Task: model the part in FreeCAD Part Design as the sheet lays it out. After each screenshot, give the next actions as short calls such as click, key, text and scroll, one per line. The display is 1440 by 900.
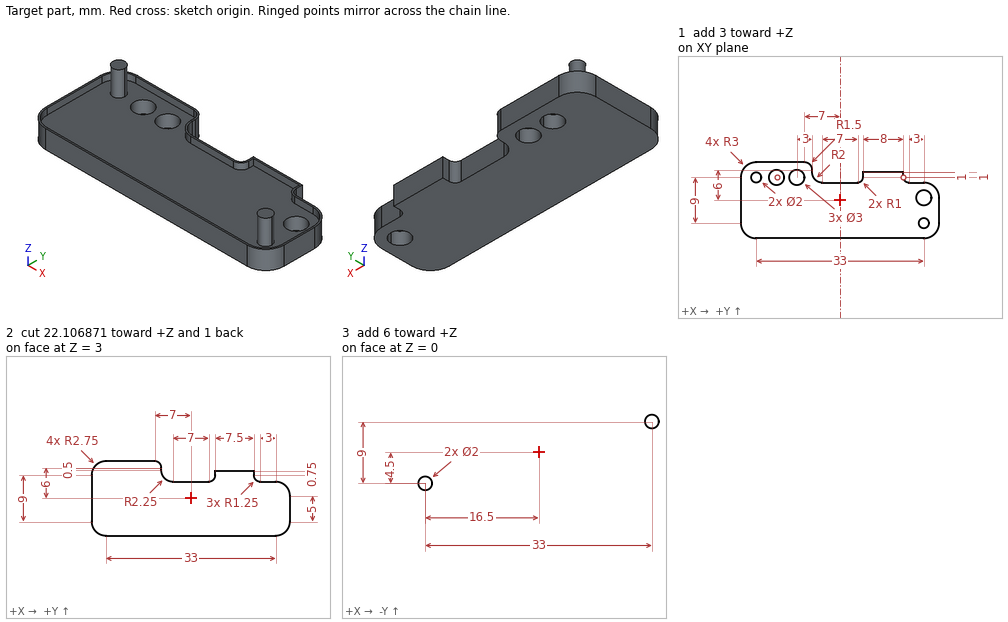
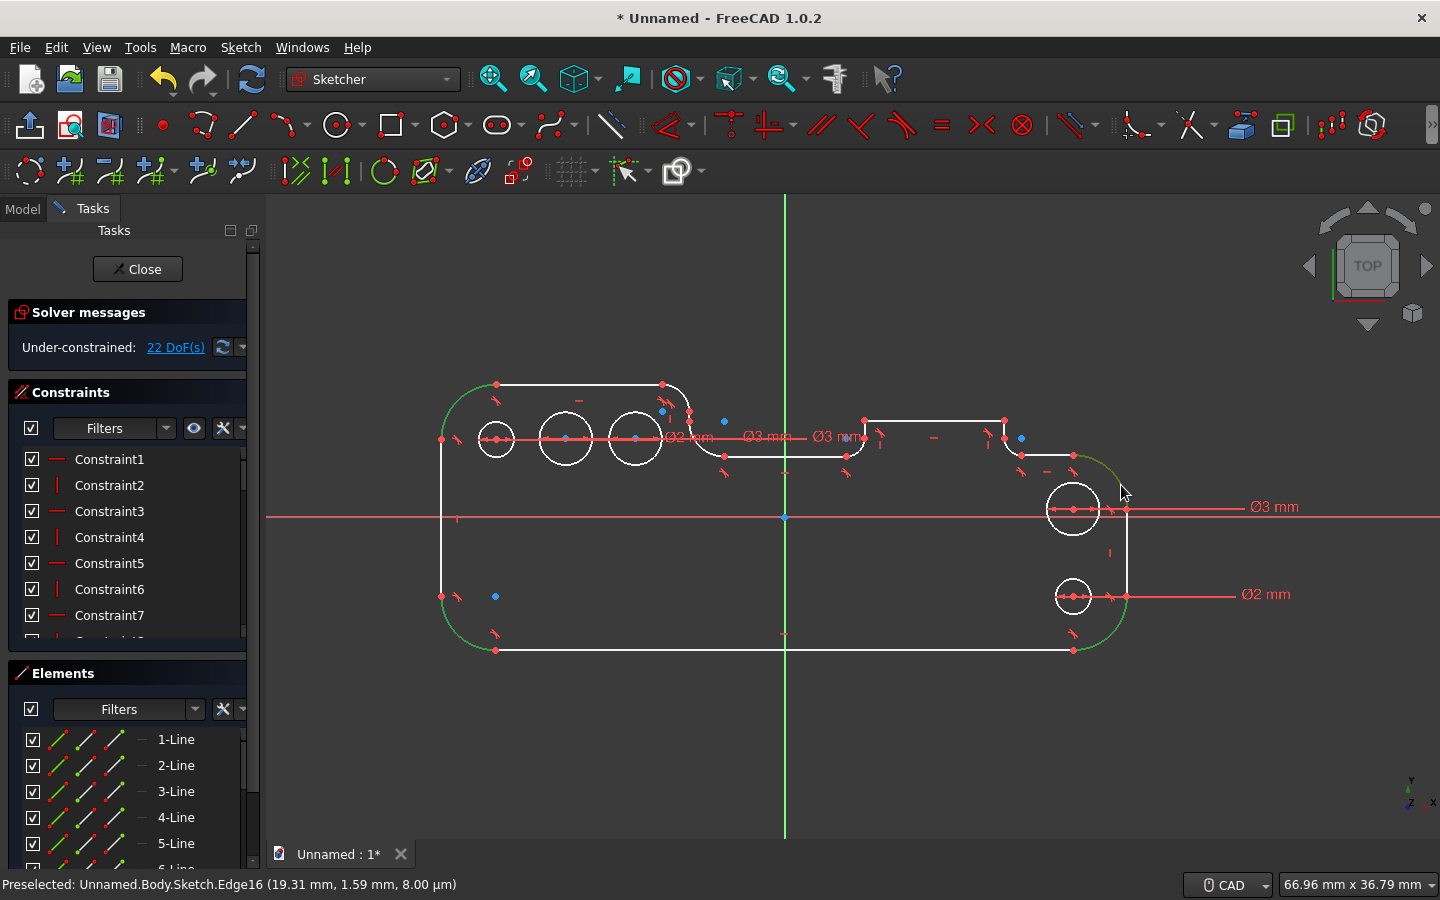
click(942, 126)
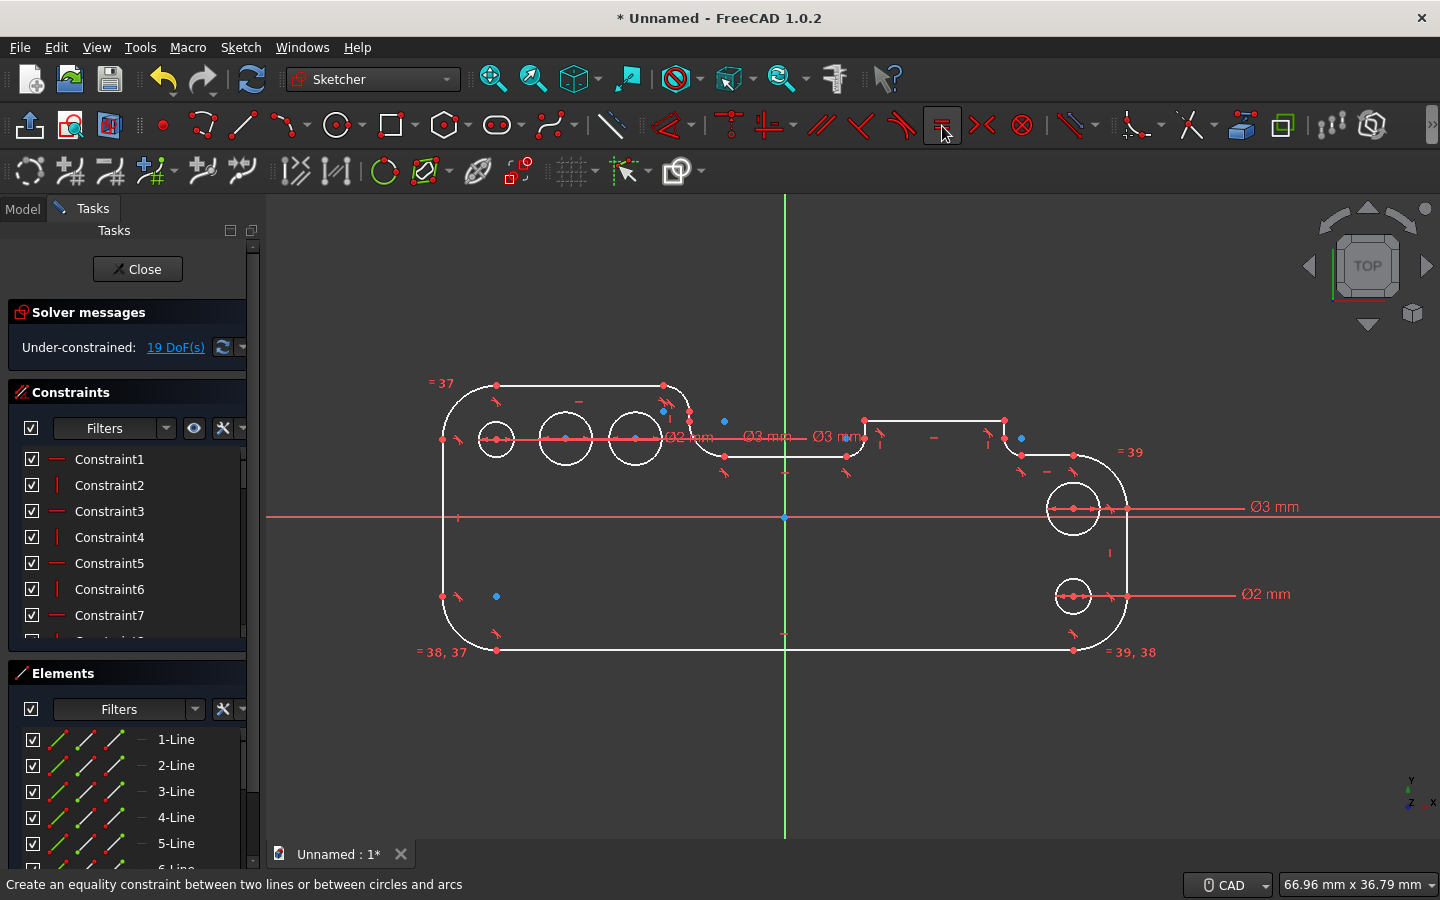
click(1009, 450)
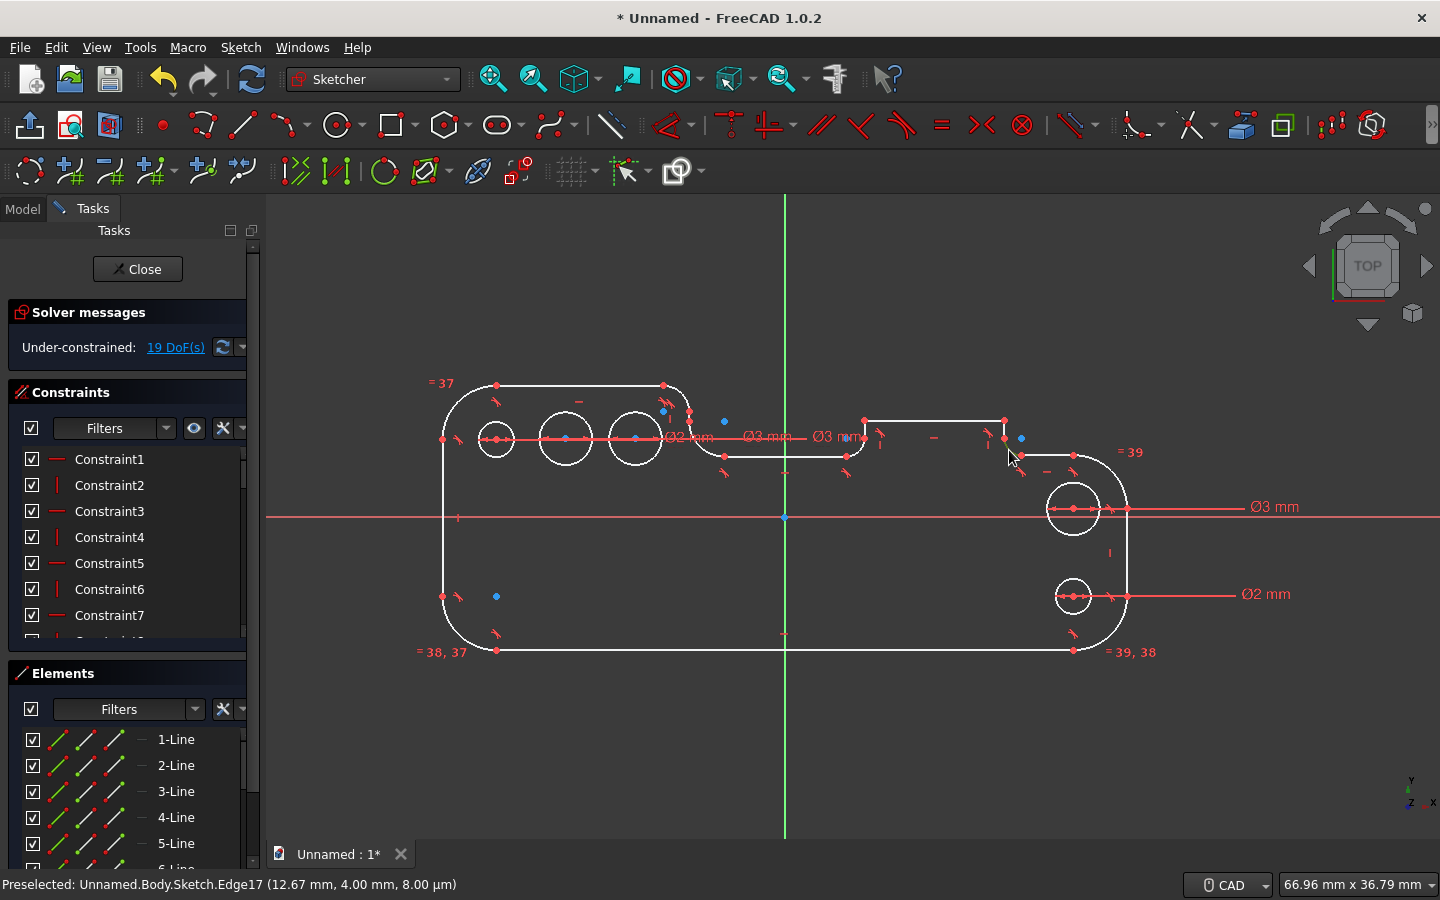
click(859, 451)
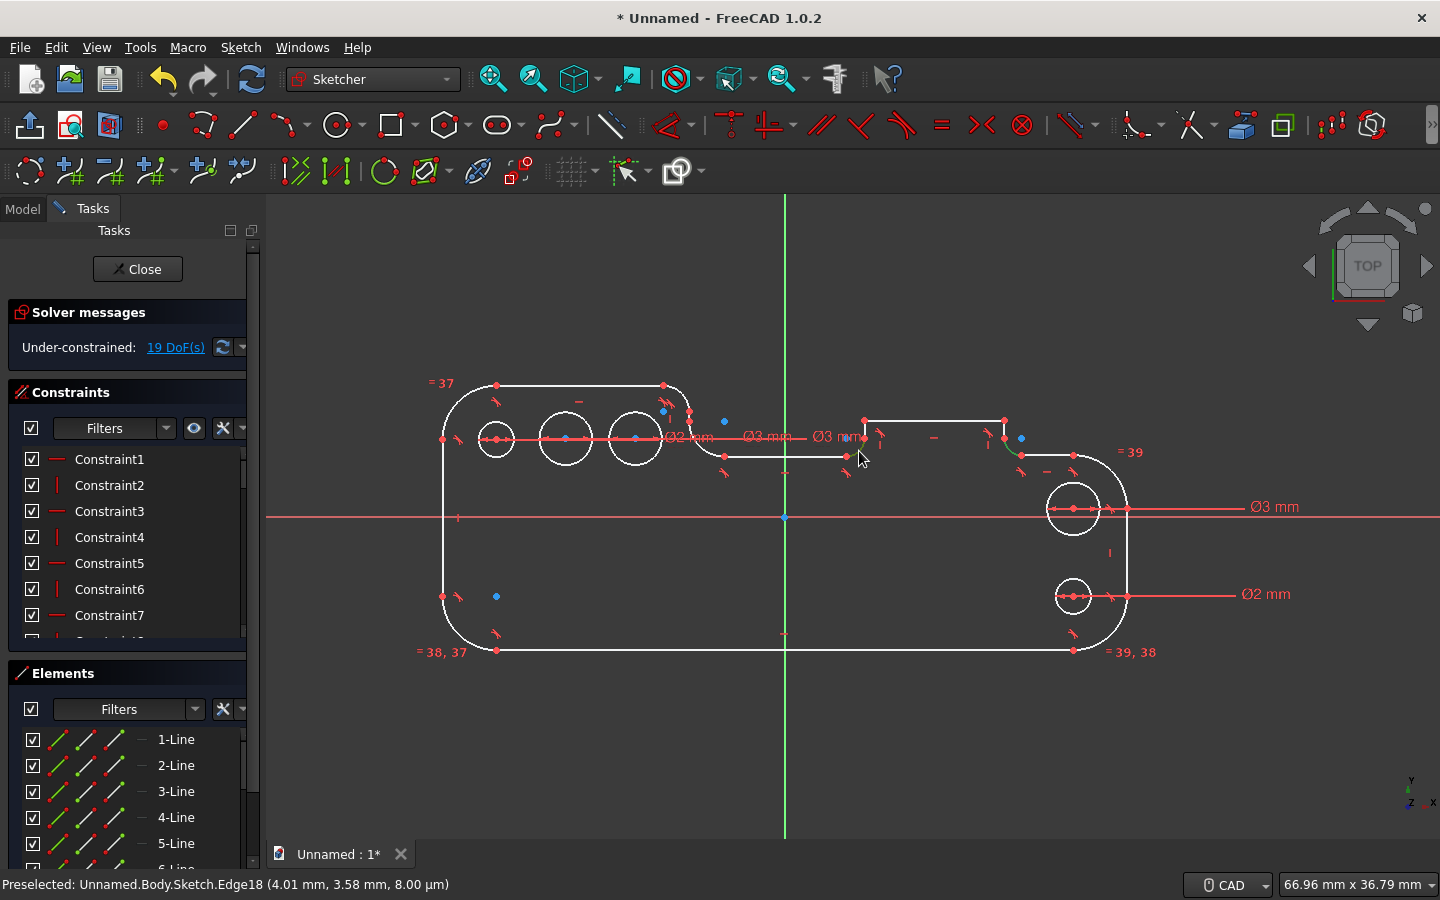
click(942, 126)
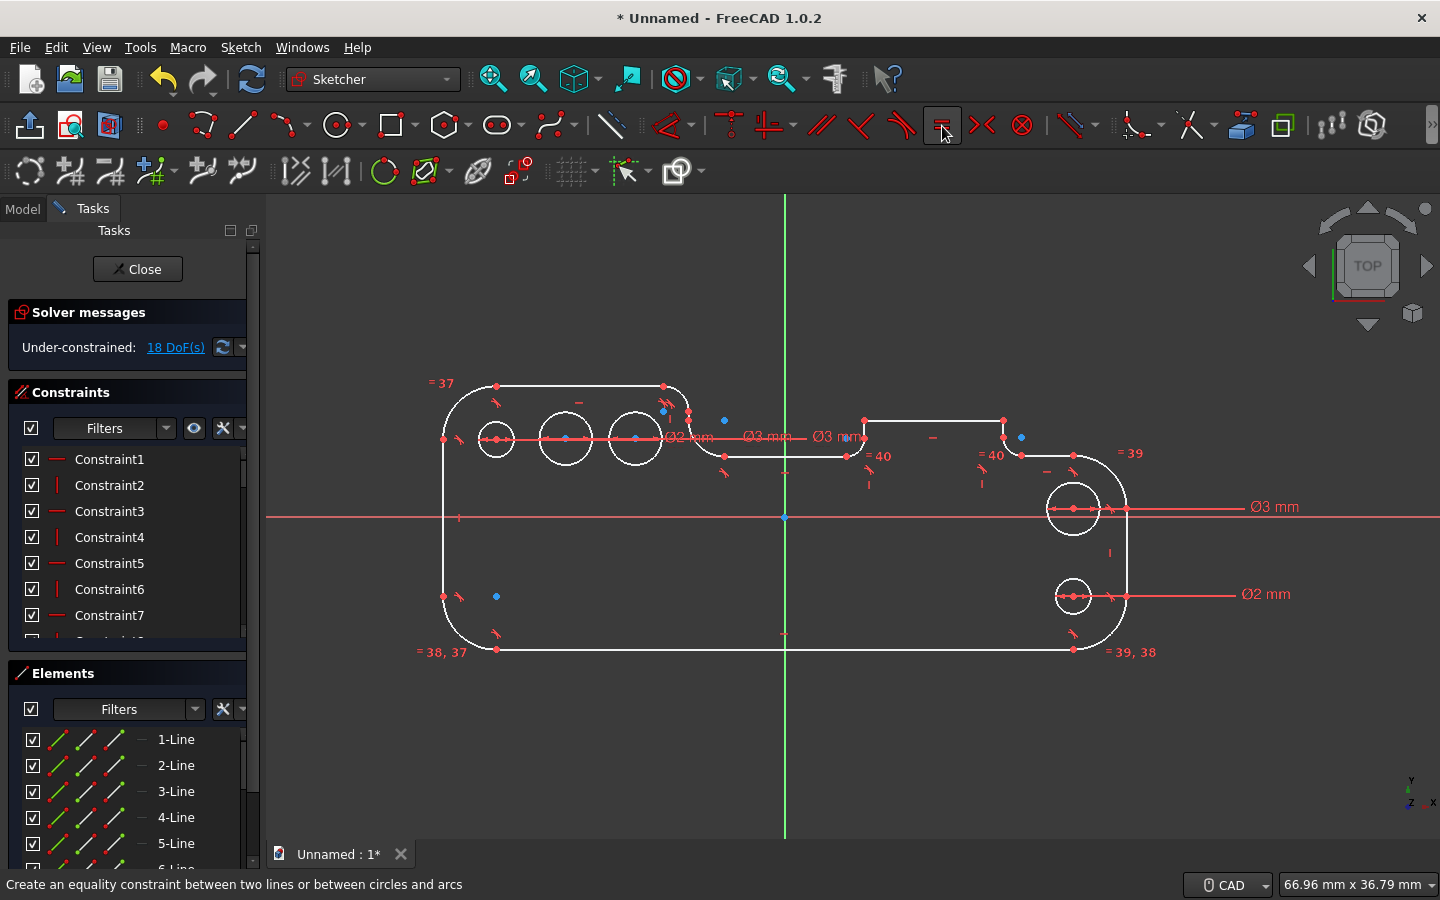
click(635, 439)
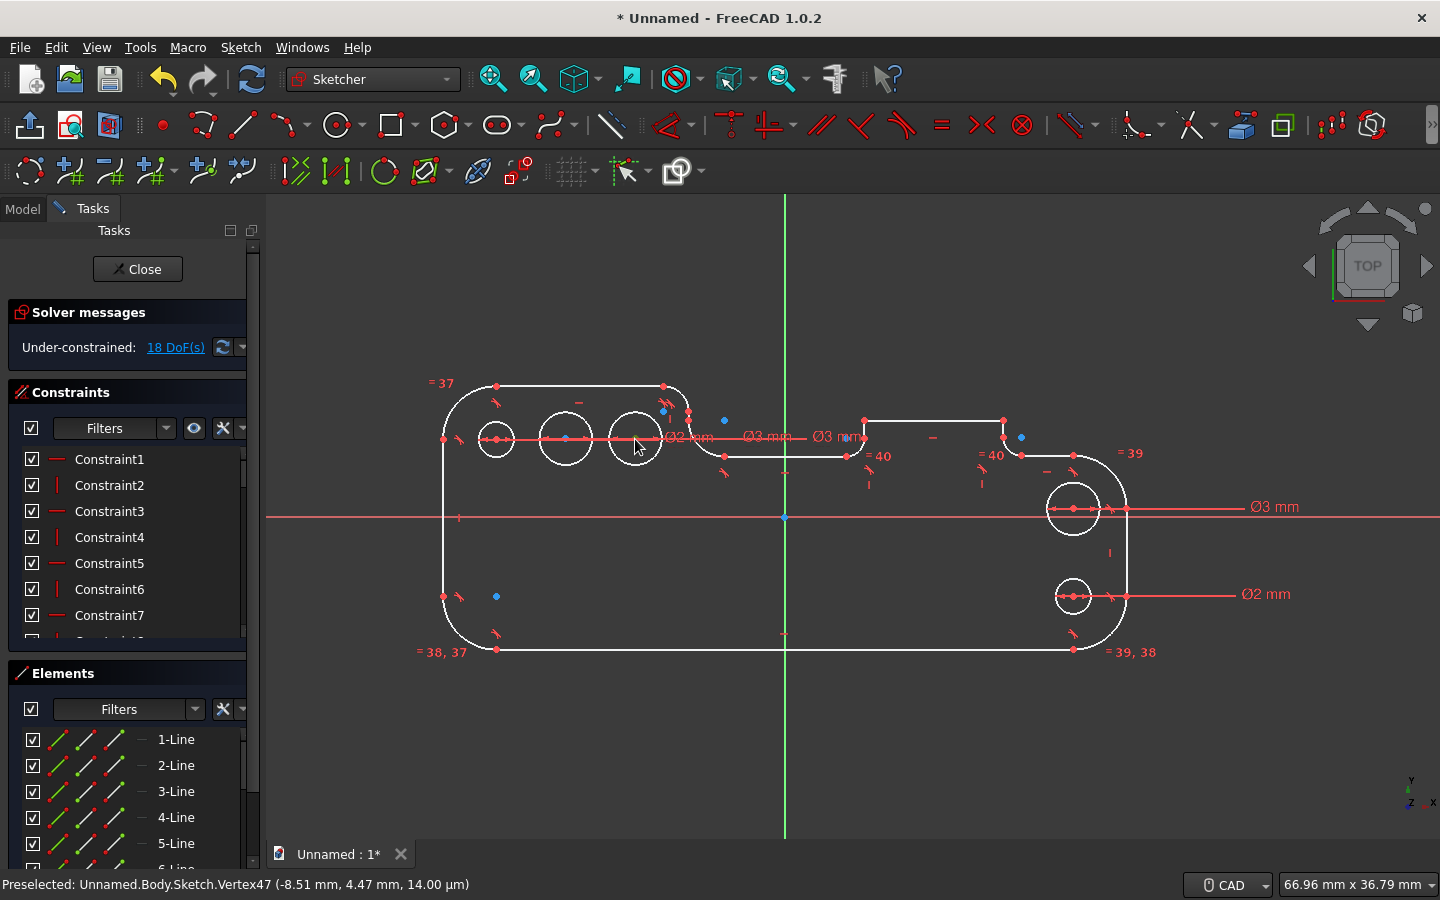
click(566, 439)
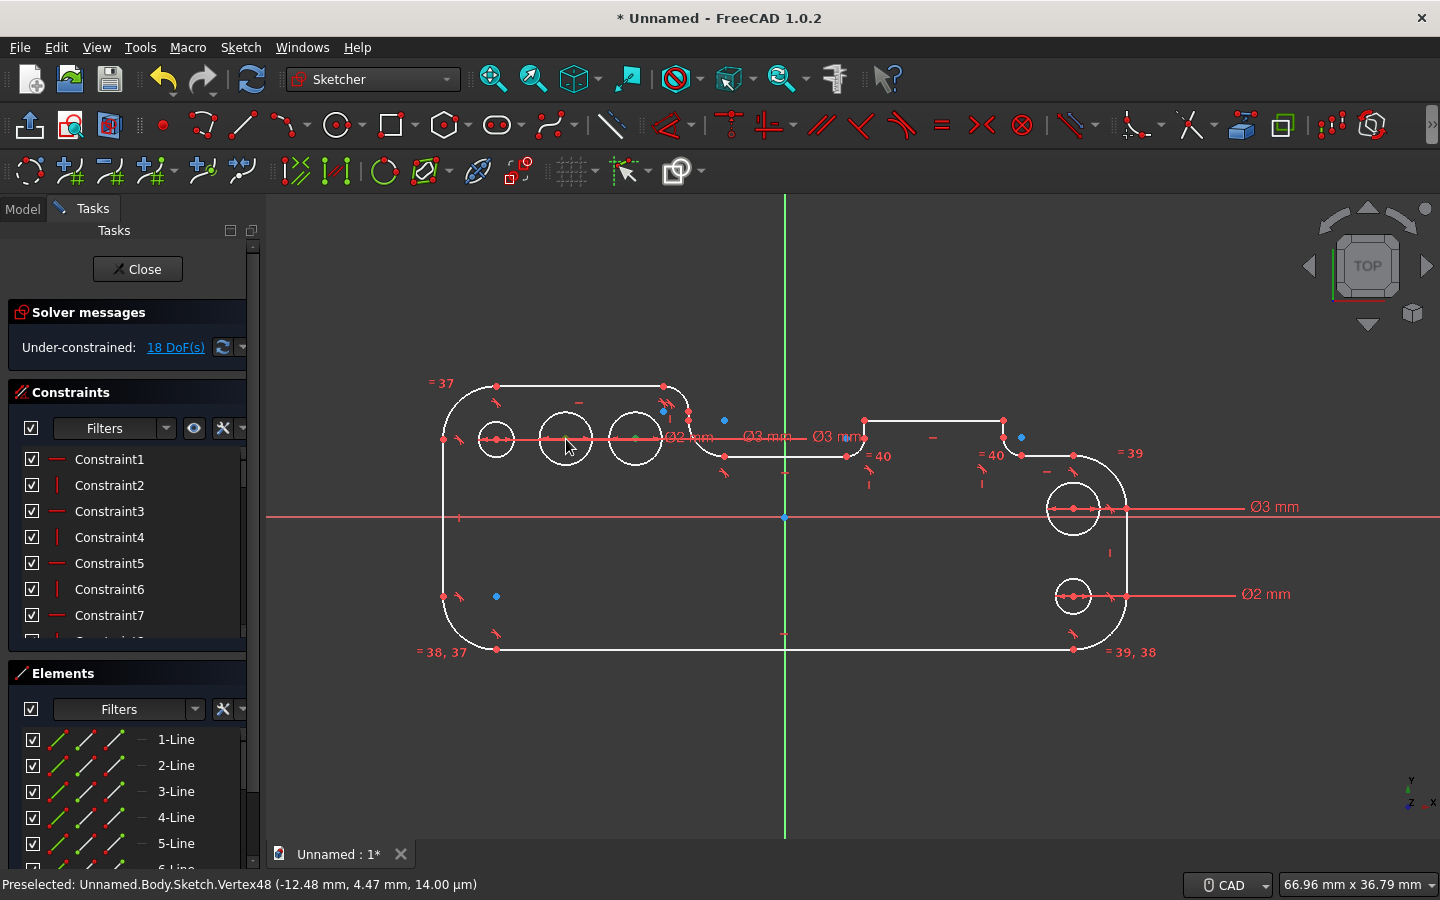
click(796, 126)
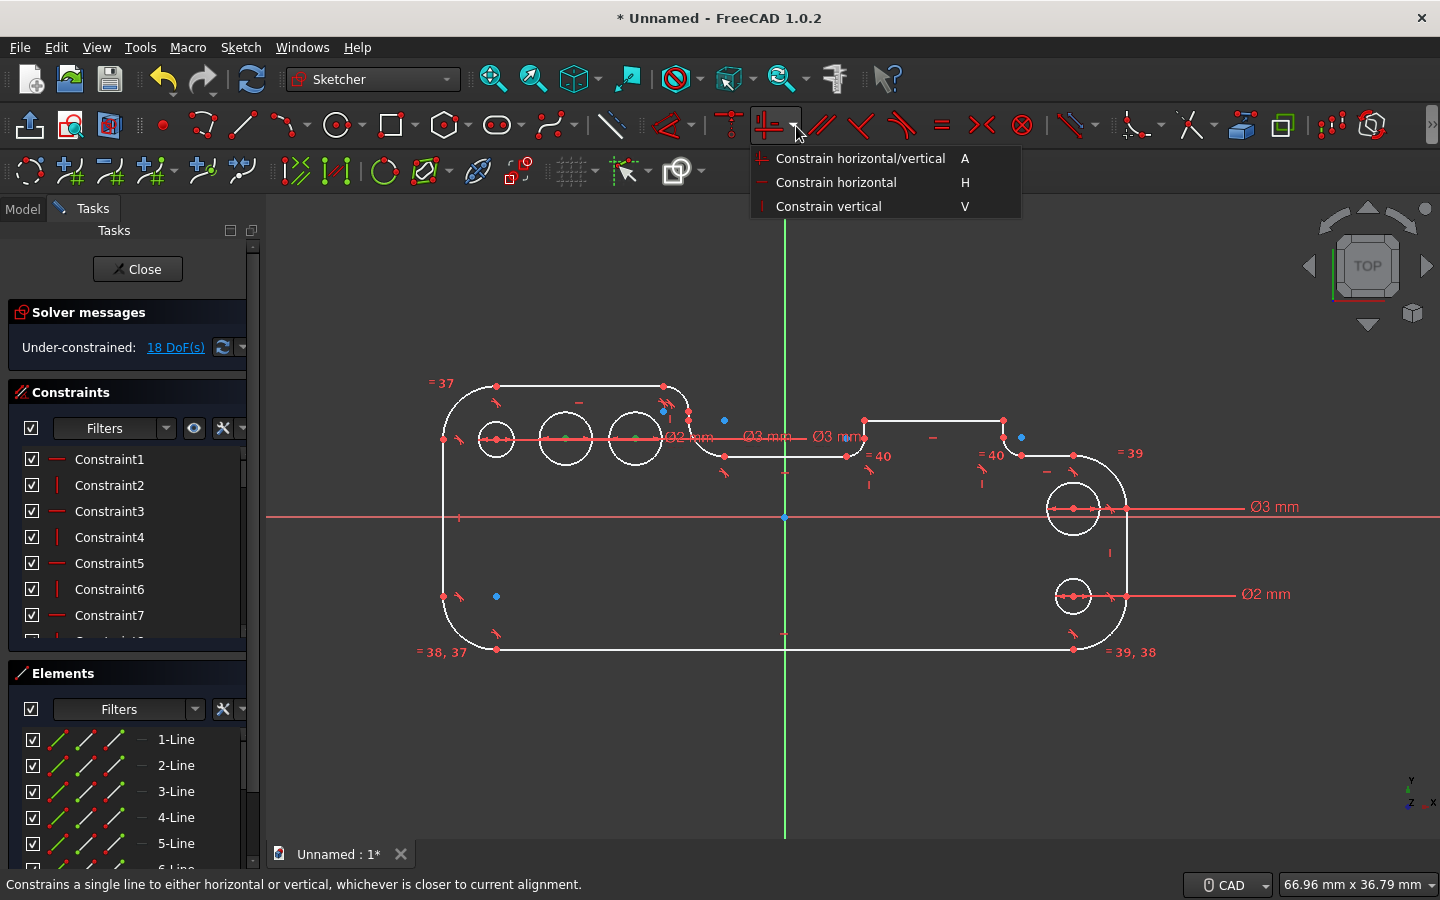
click(886, 182)